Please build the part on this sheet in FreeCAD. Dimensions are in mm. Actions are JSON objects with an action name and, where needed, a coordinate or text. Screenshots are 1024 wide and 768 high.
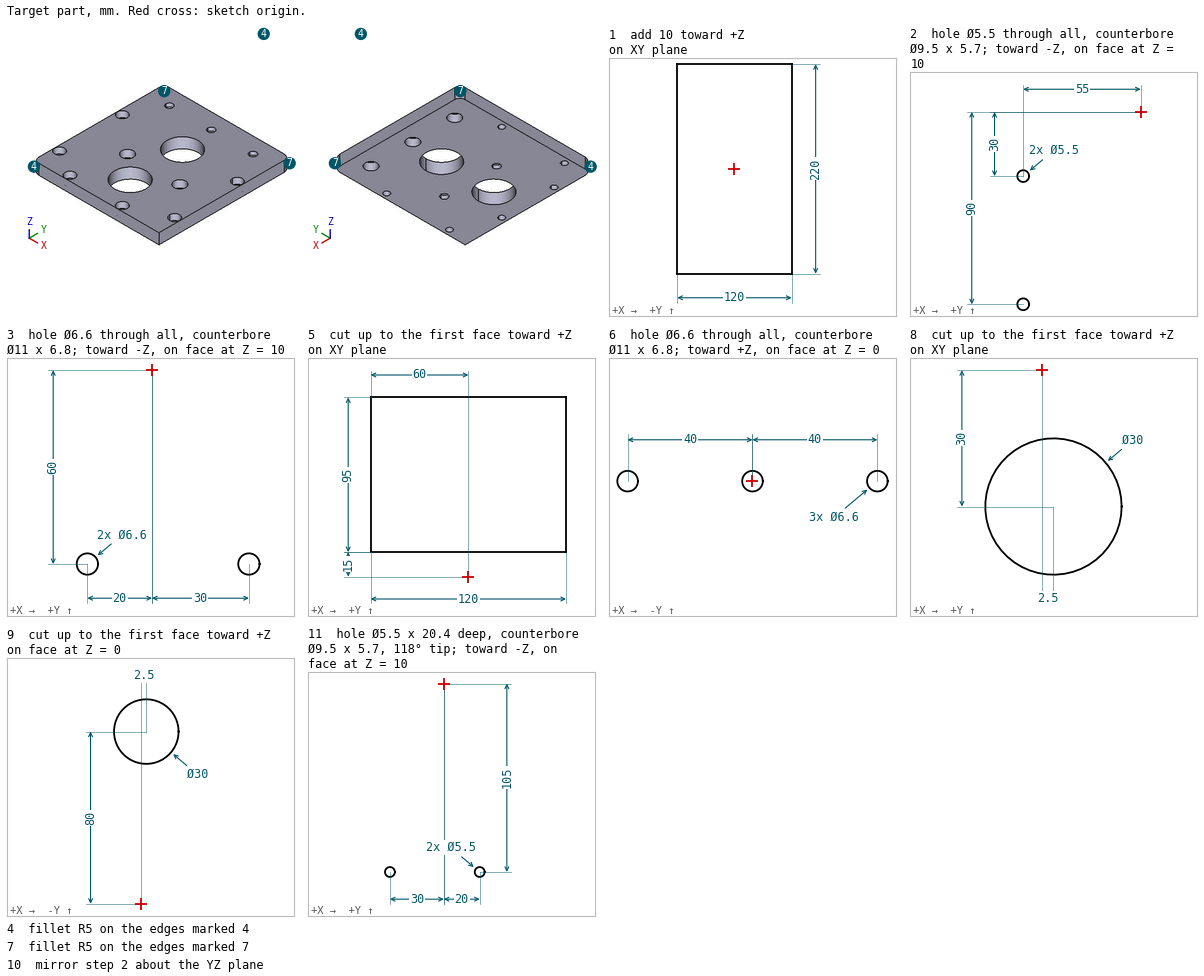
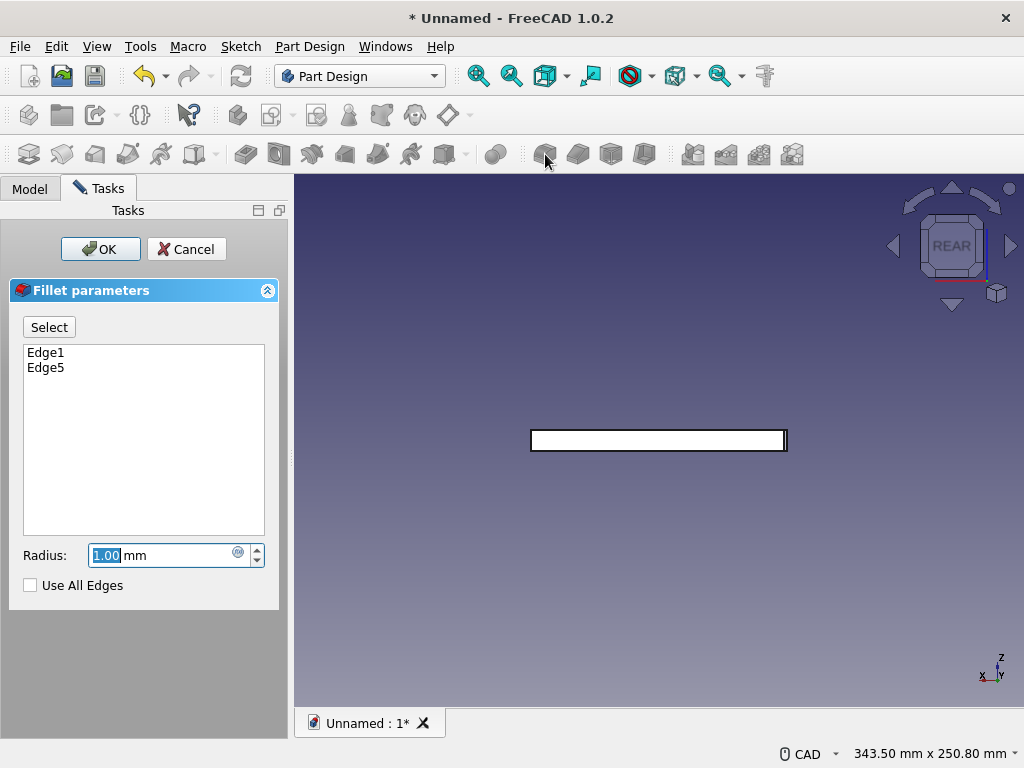
{"action": "type", "text": "5"}
{"action": "key", "text": "Tab"}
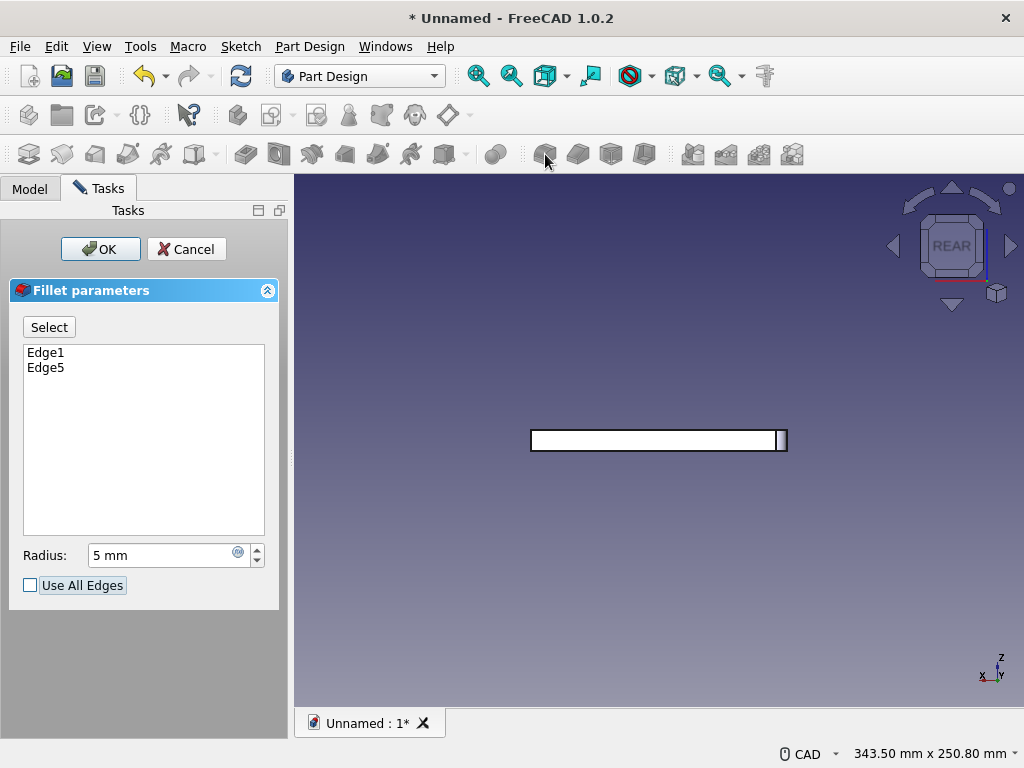
{"action": "left_click", "coordinate": [101, 249]}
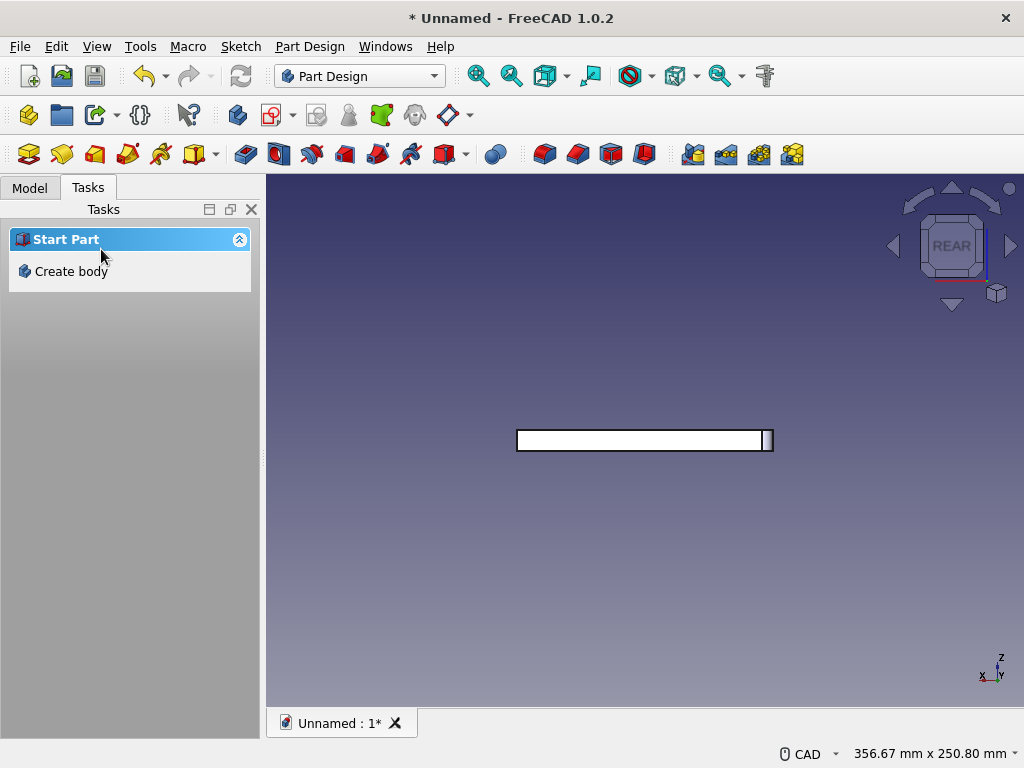
{"action": "left_click", "coordinate": [479, 76]}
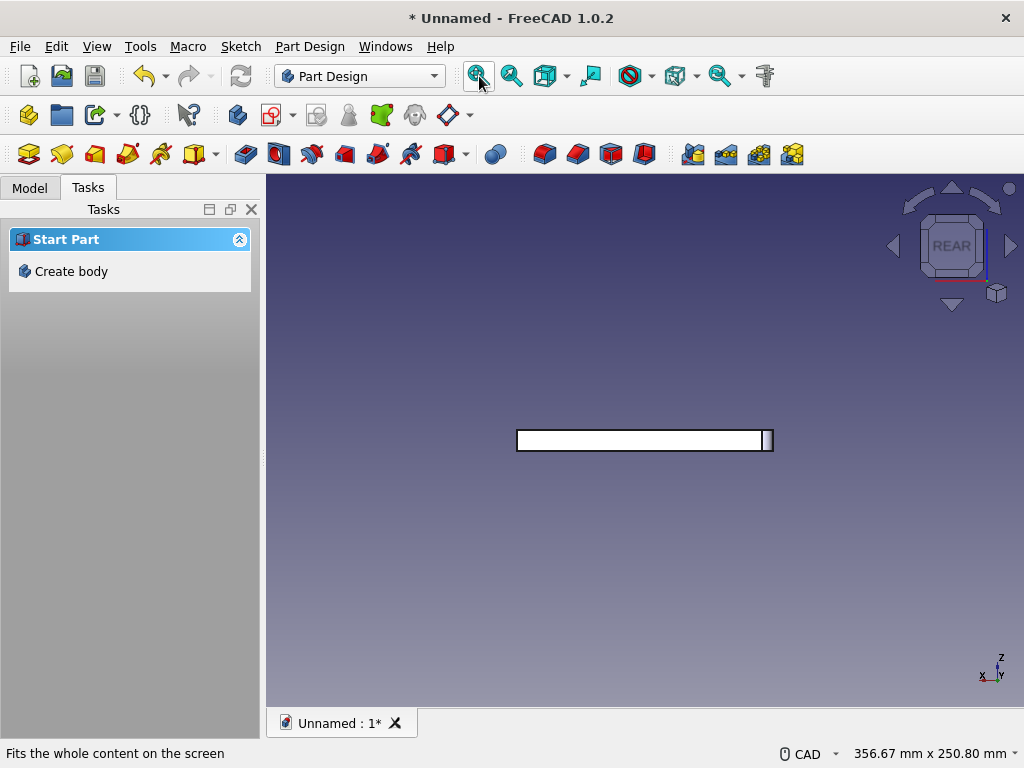
{"action": "left_click", "coordinate": [270, 116]}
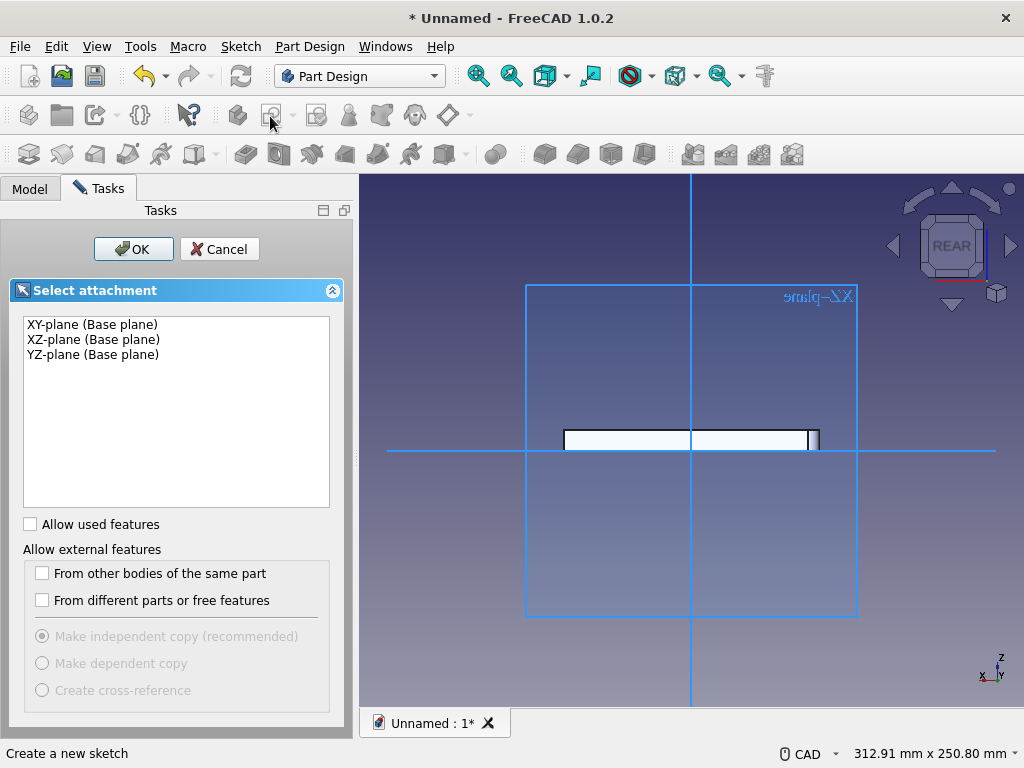
{"action": "left_click", "coordinate": [84, 324]}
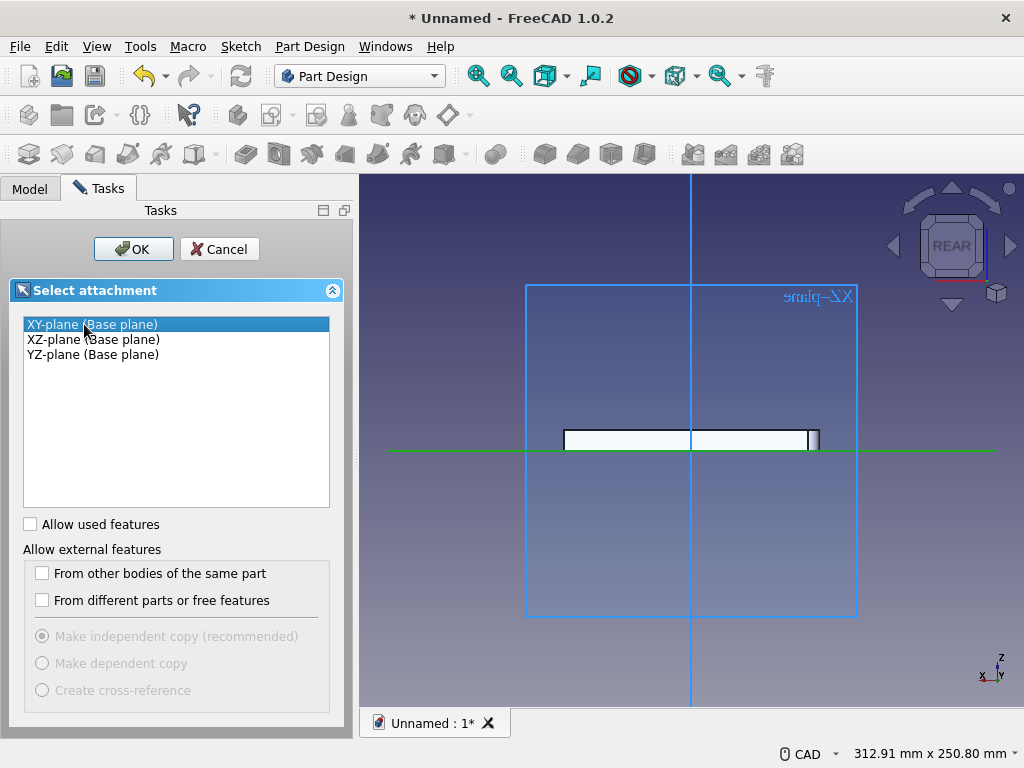
{"action": "left_click", "coordinate": [134, 249]}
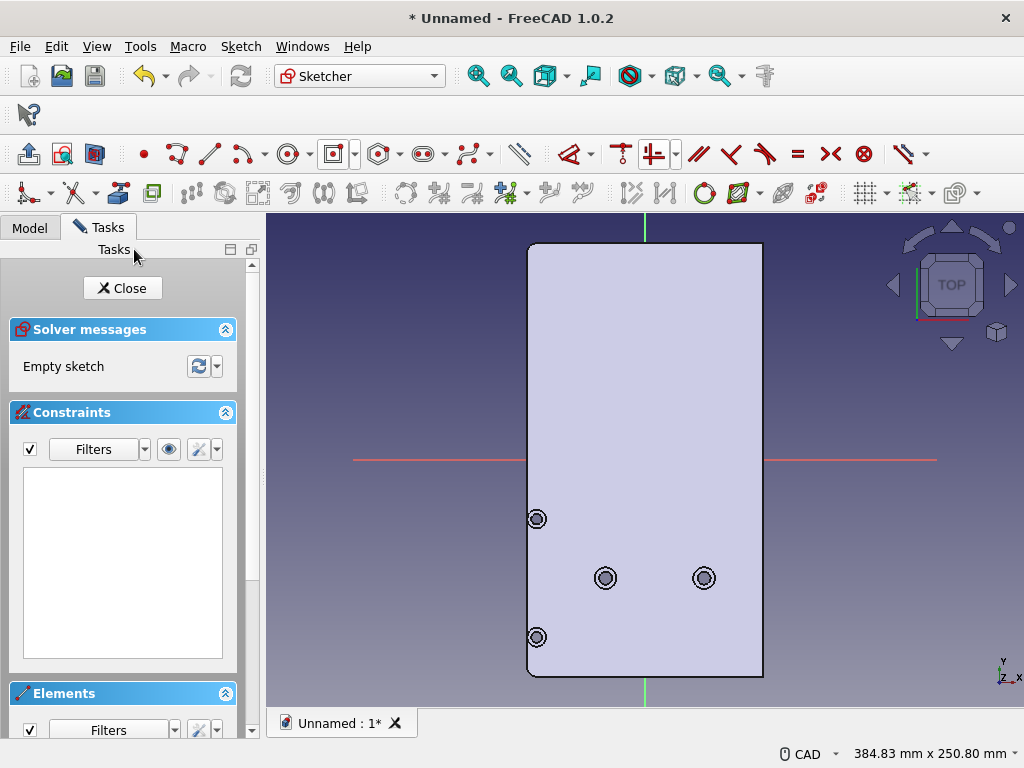
{"action": "left_click", "coordinate": [95, 154]}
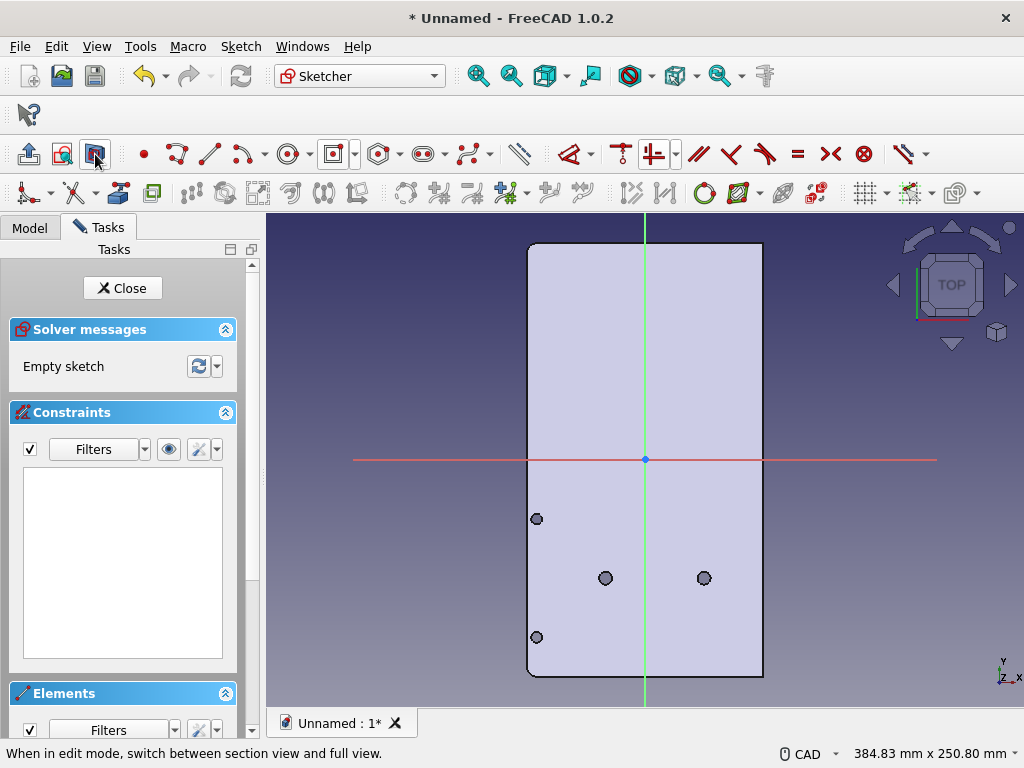
{"action": "scroll", "coordinate": [294, 679], "scroll_direction": "down", "scroll_amount": 1}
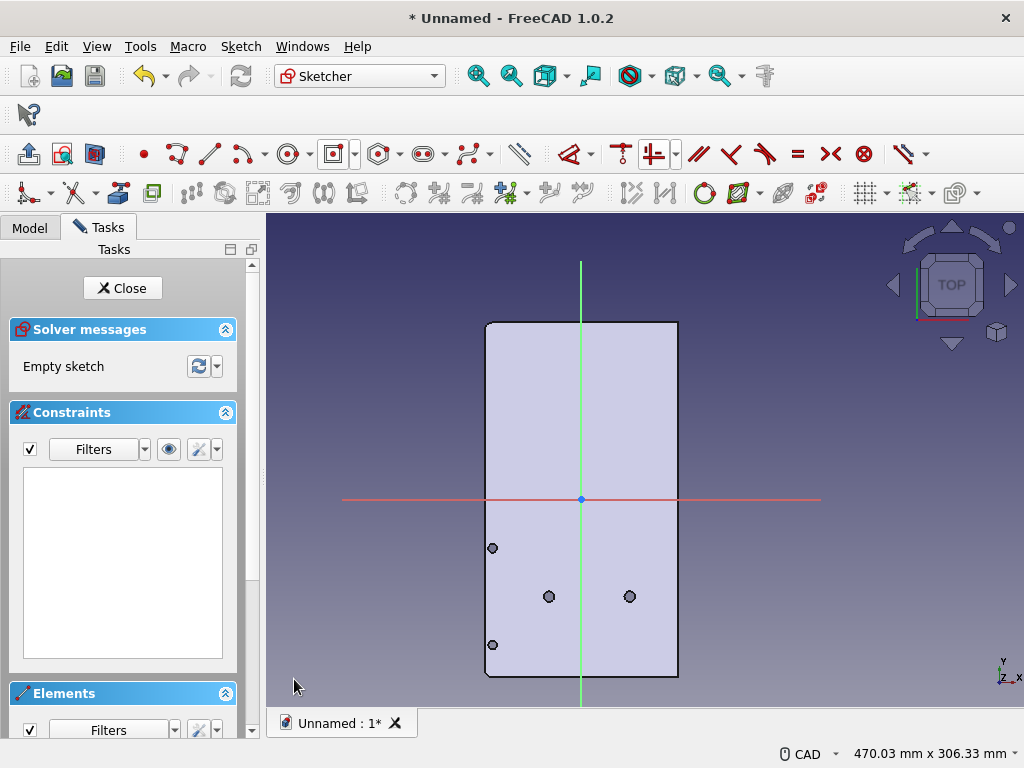
{"action": "scroll", "coordinate": [587, 352], "scroll_direction": "up", "scroll_amount": 3}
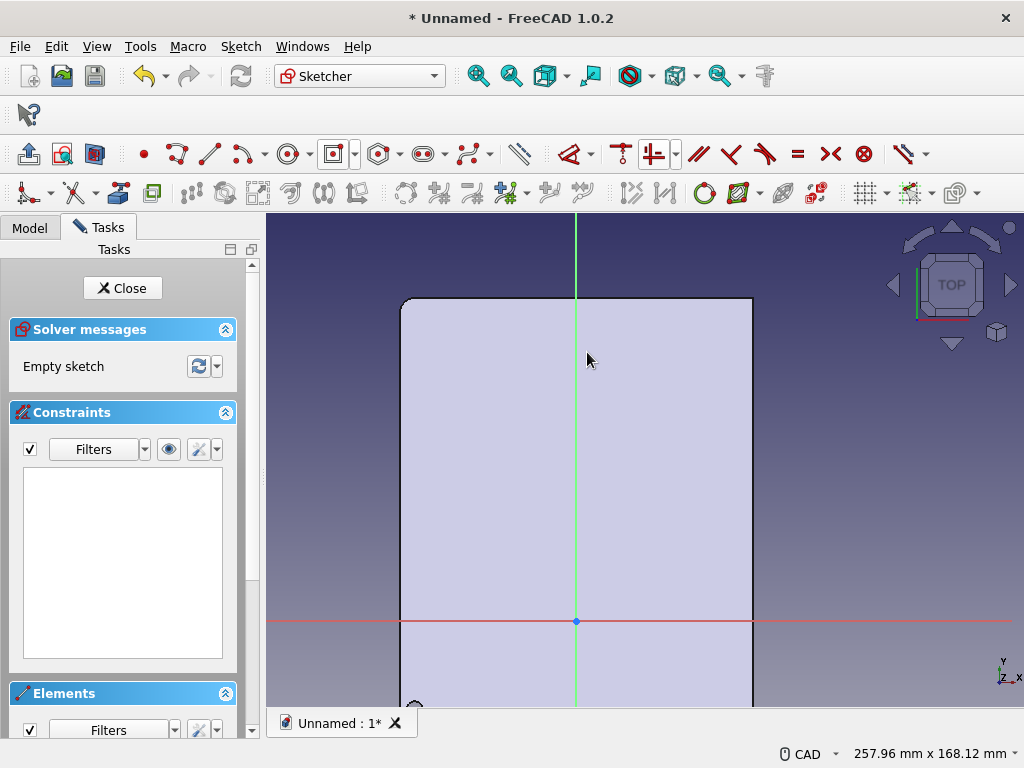
{"action": "key", "text": "g r"}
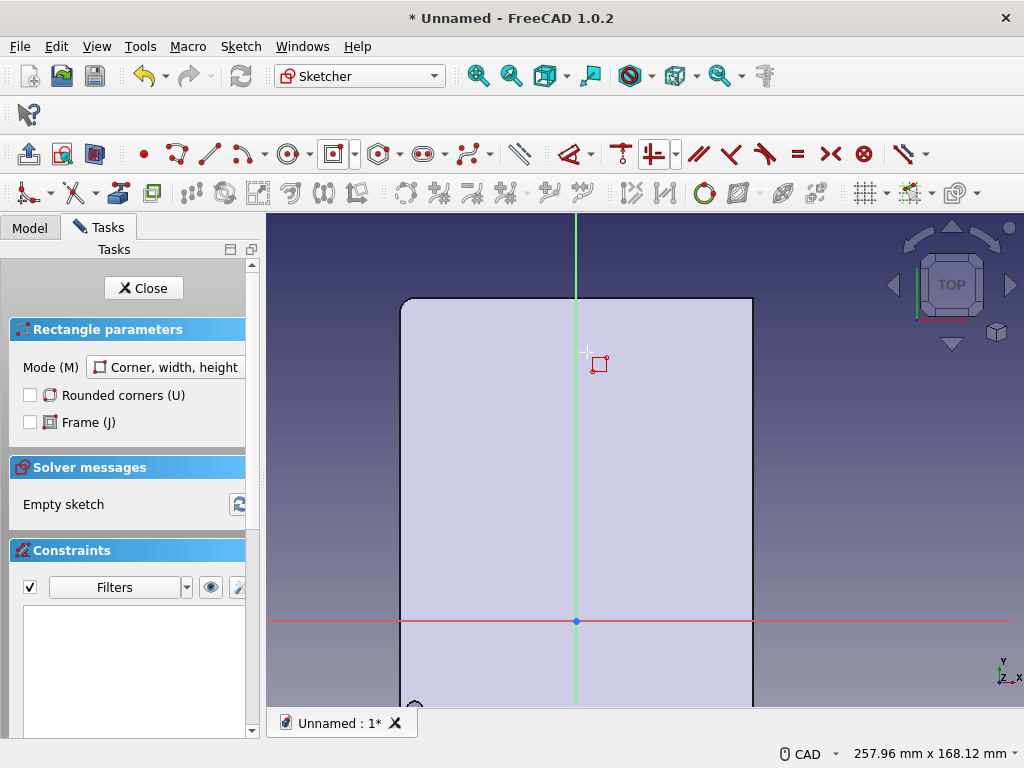
{"action": "left_click", "coordinate": [400, 298]}
{"action": "left_click", "coordinate": [753, 577]}
{"action": "key", "text": "Escape"}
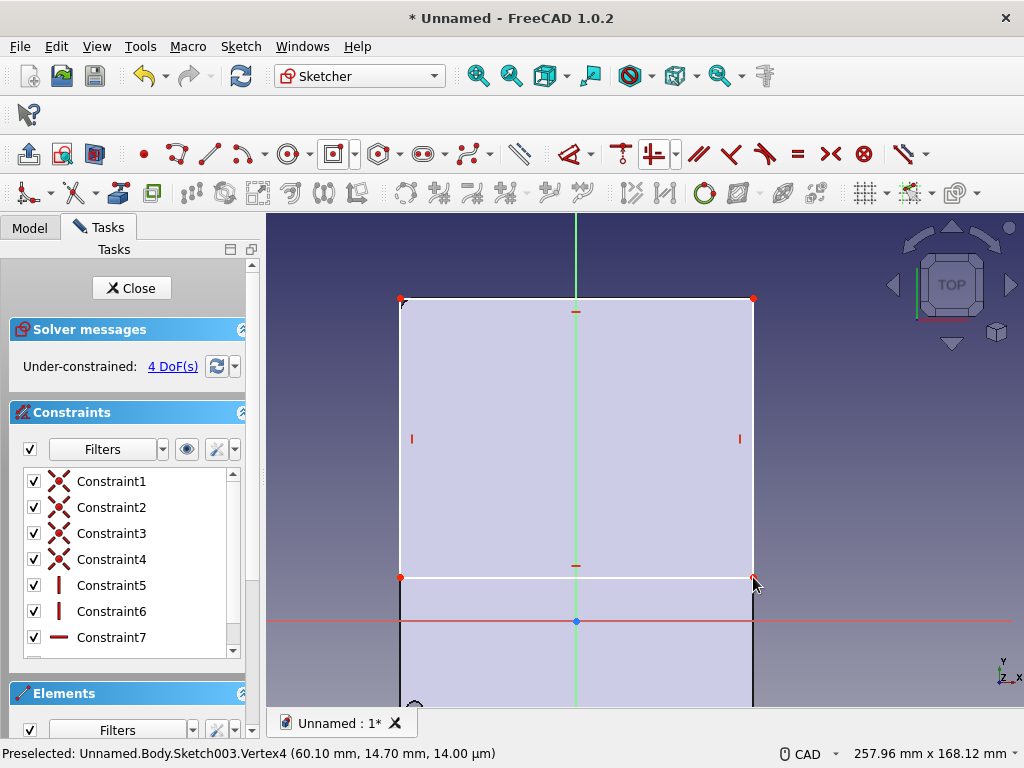
{"action": "left_click", "coordinate": [568, 154]}